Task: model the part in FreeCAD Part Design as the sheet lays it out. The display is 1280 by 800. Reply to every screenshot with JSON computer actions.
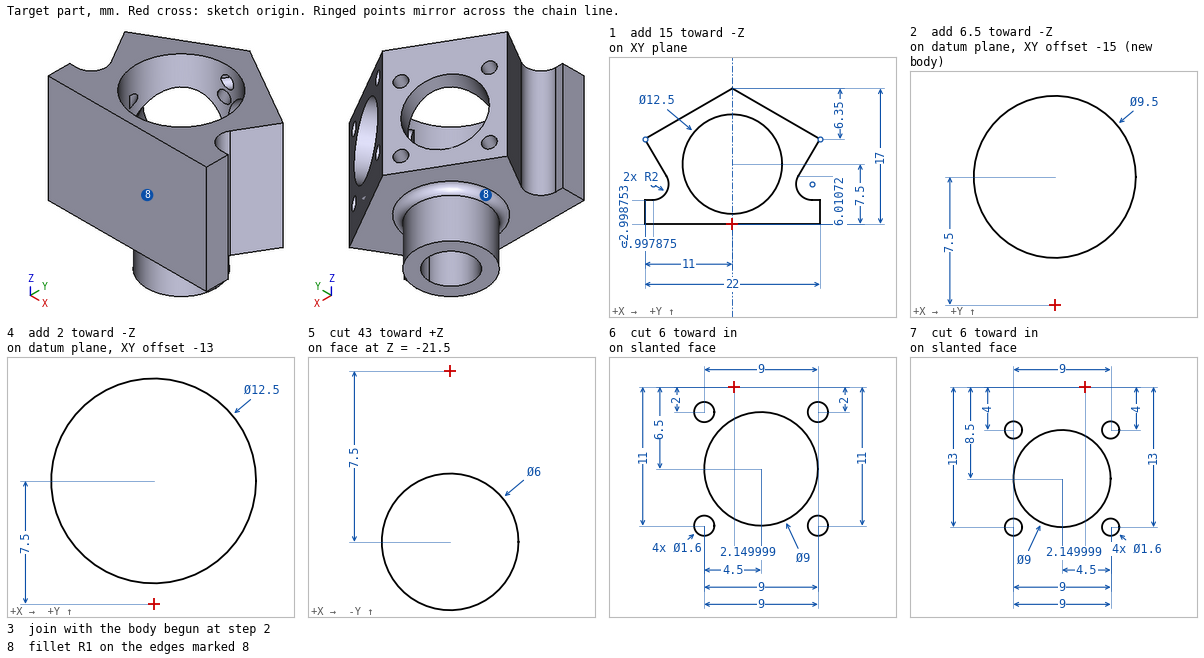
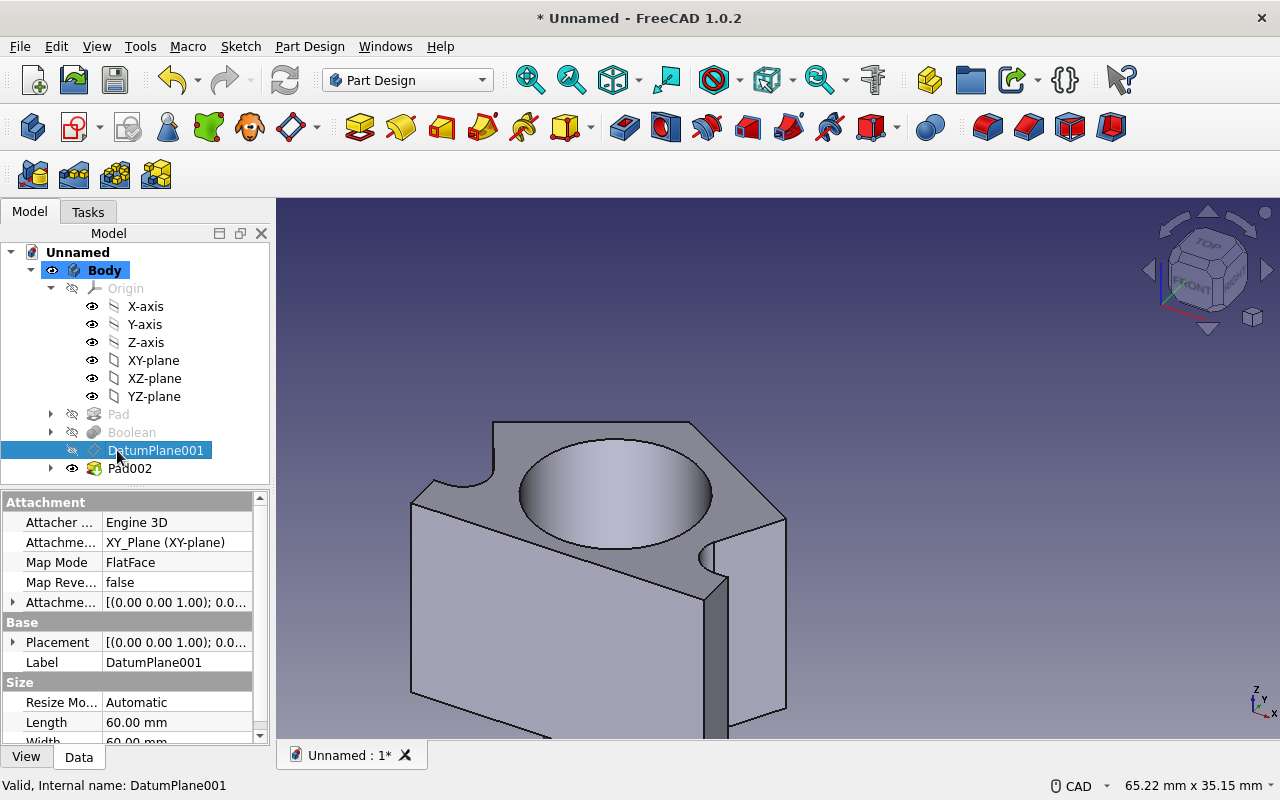
{"action": "left_click", "coordinate": [531, 80]}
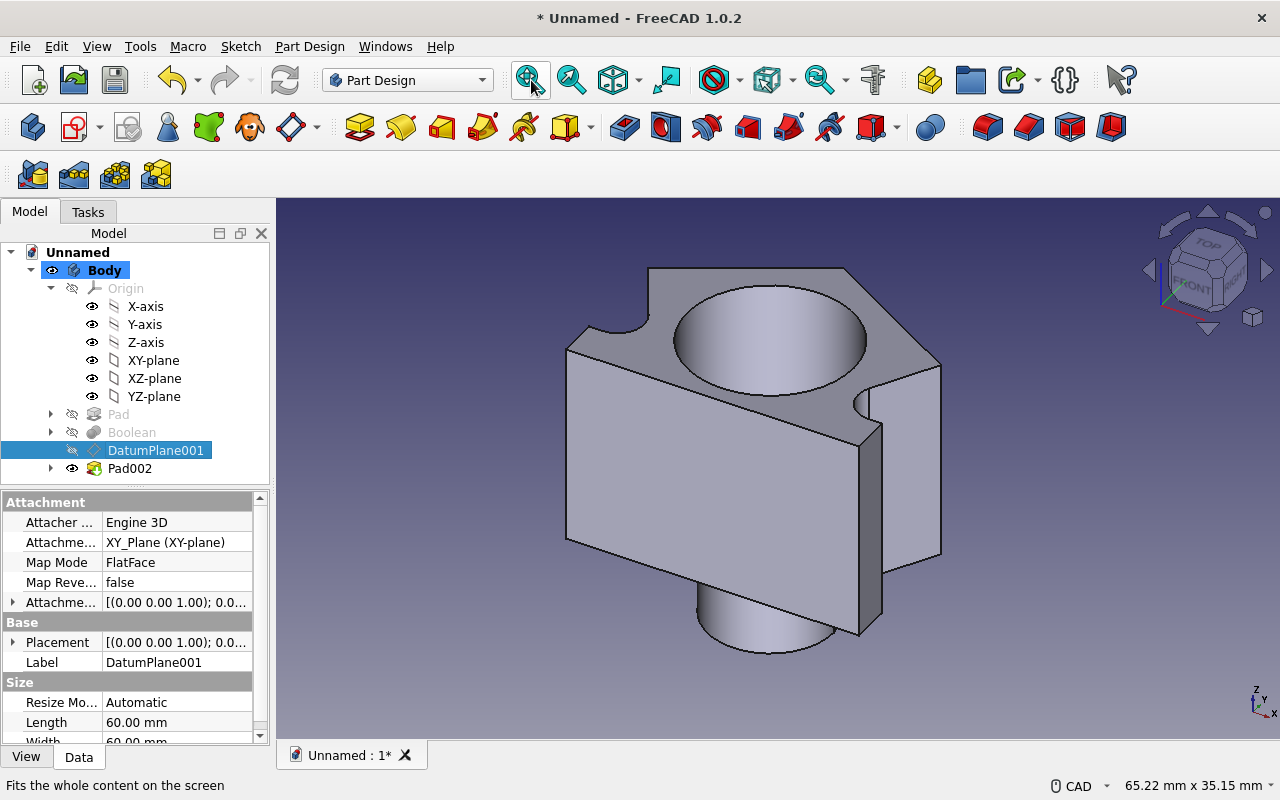
{"action": "key", "text": "5"}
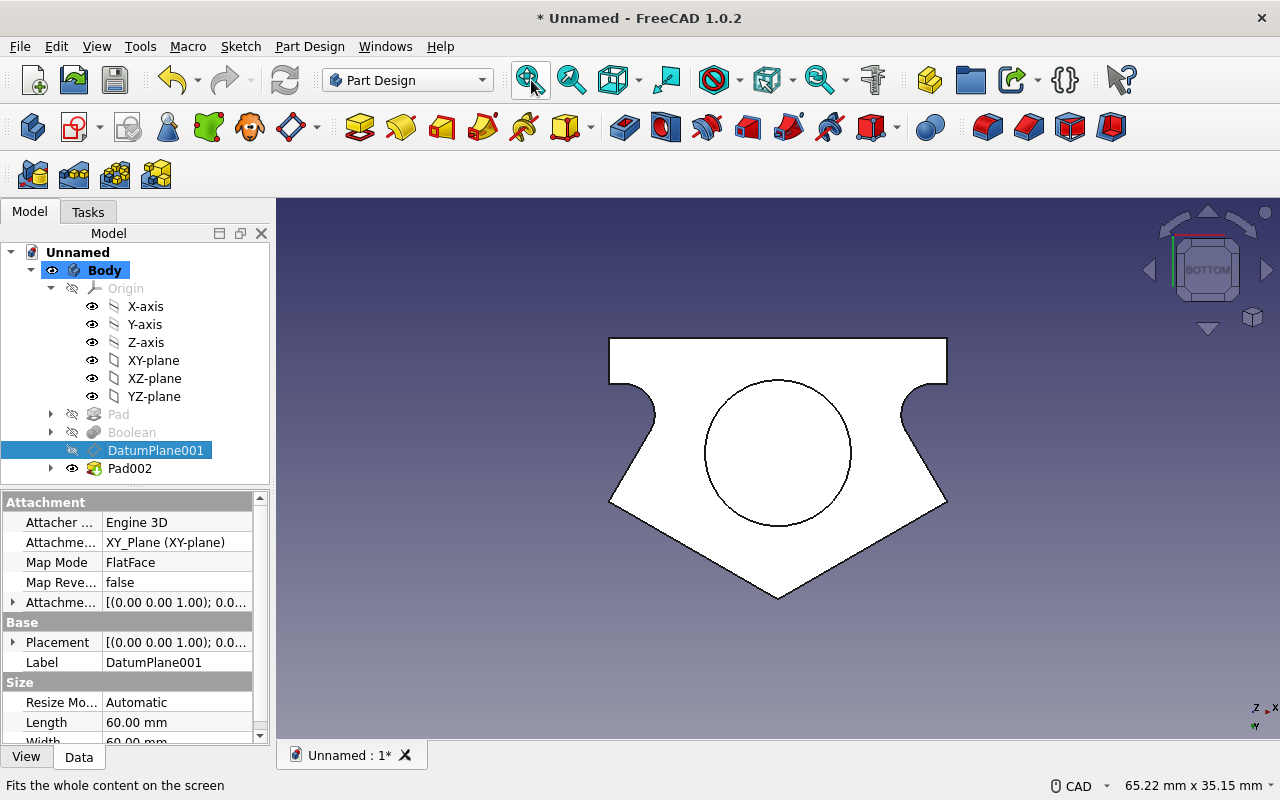
{"action": "left_click", "coordinate": [778, 452]}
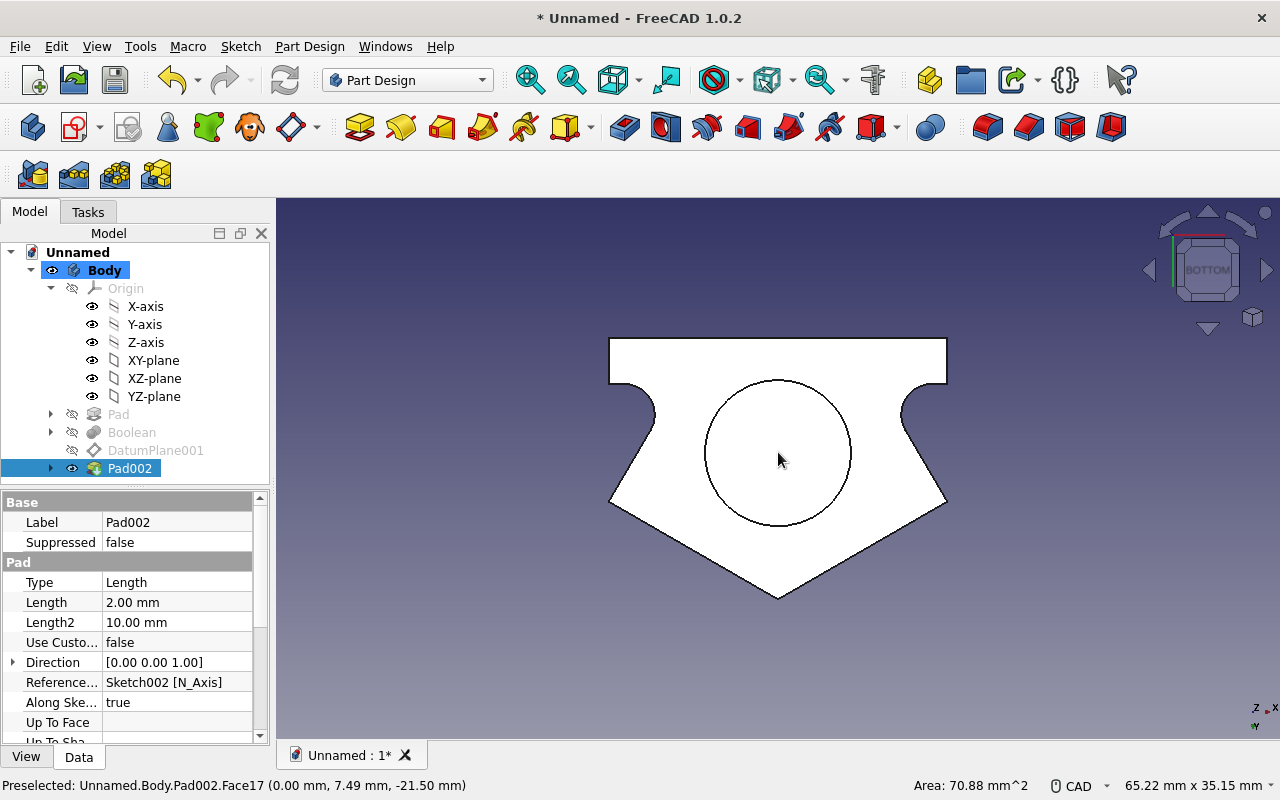
{"action": "left_click", "coordinate": [74, 128]}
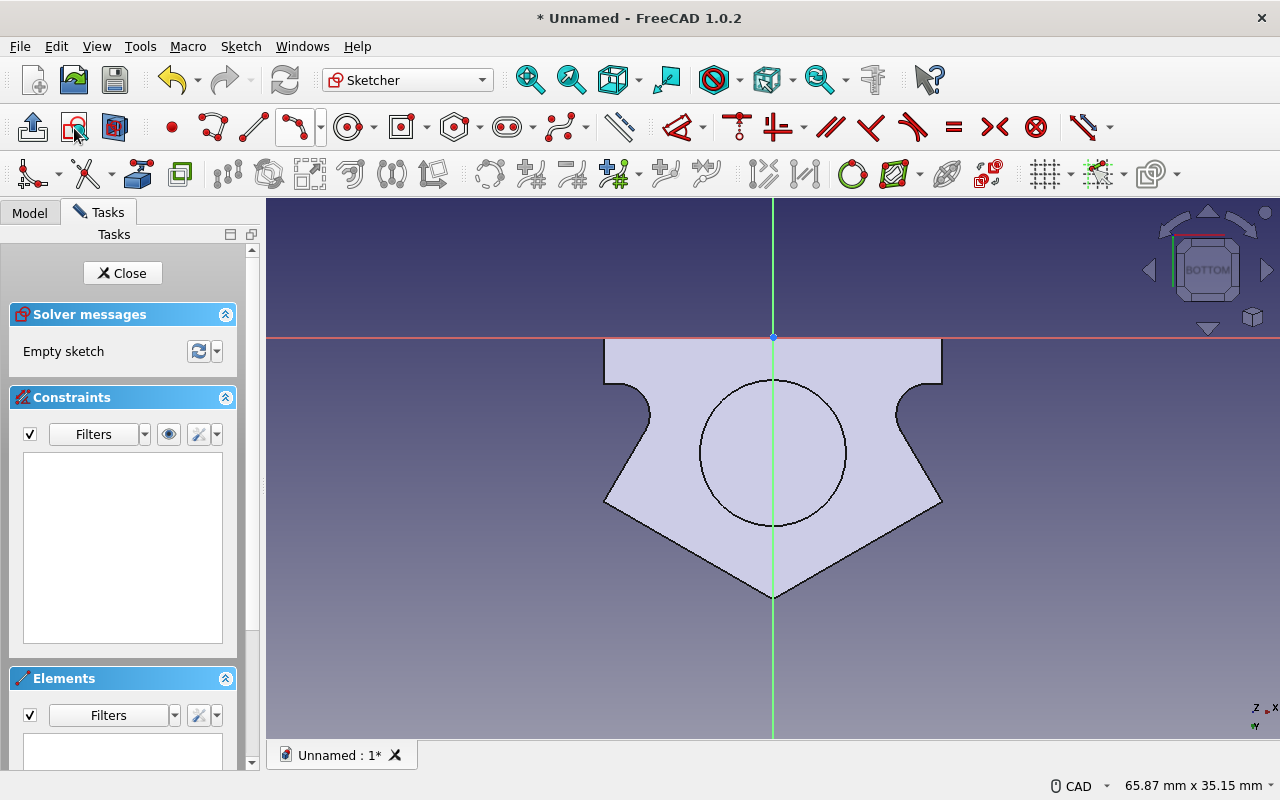
{"action": "scroll", "coordinate": [829, 378], "scroll_direction": "up", "scroll_amount": 4}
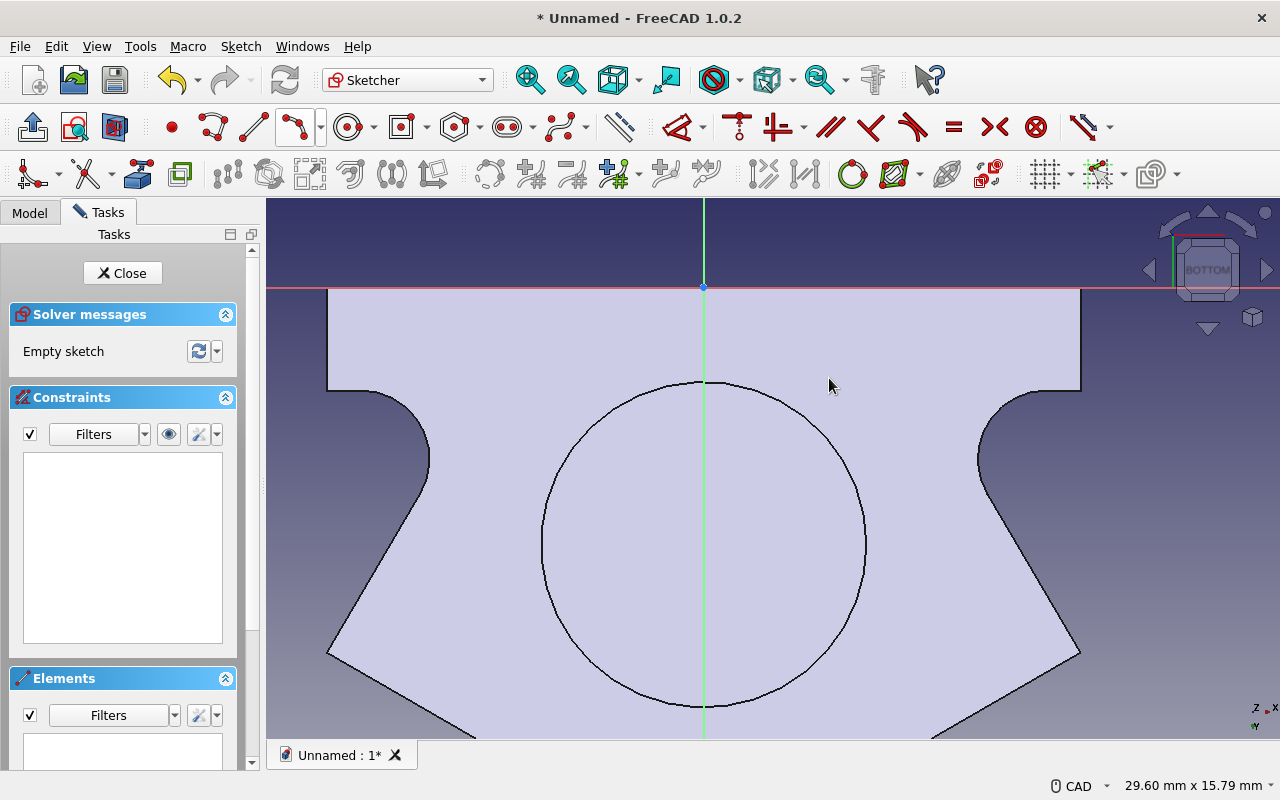
{"action": "left_click", "coordinate": [348, 128]}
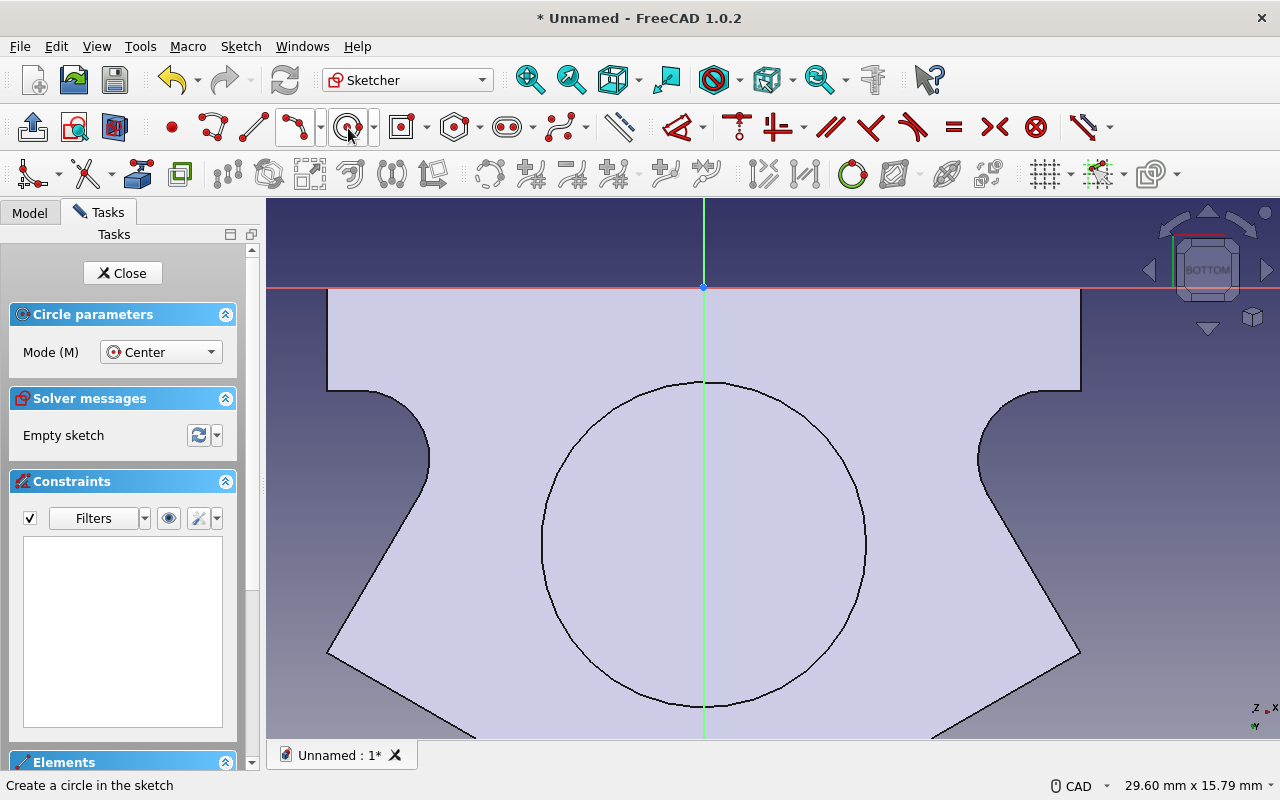
{"action": "left_click", "coordinate": [704, 545]}
{"action": "mouse_move", "coordinate": [776, 472]}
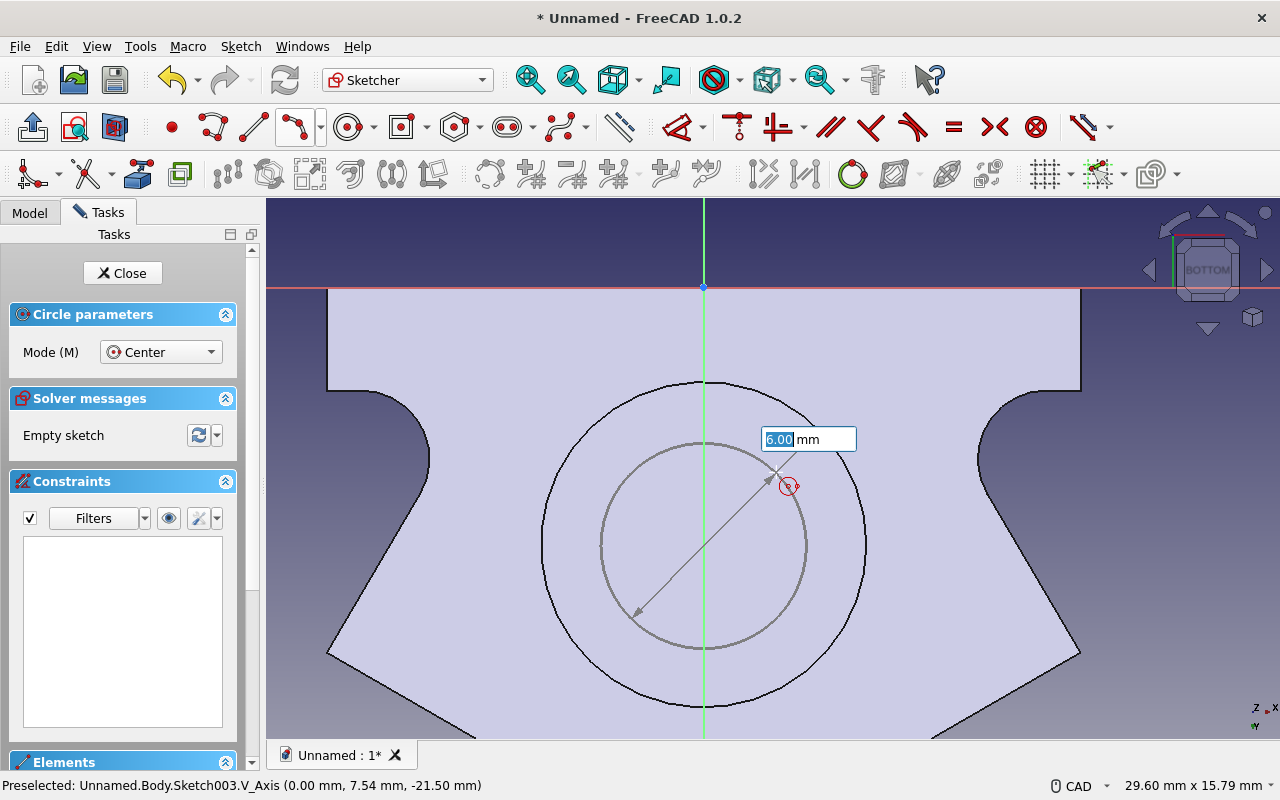
{"action": "type", "text": "6"}
{"action": "key", "text": "Return"}
{"action": "key", "text": "Escape"}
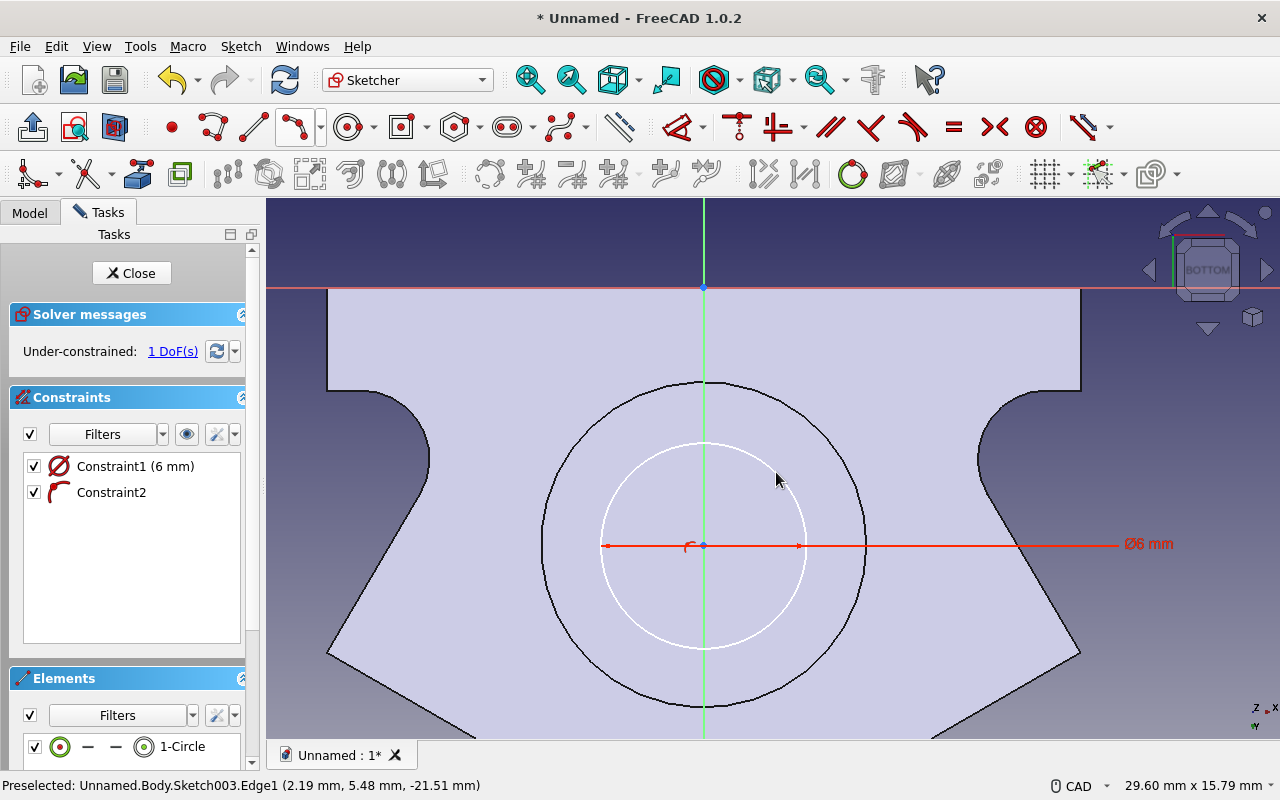
{"action": "left_click", "coordinate": [676, 128]}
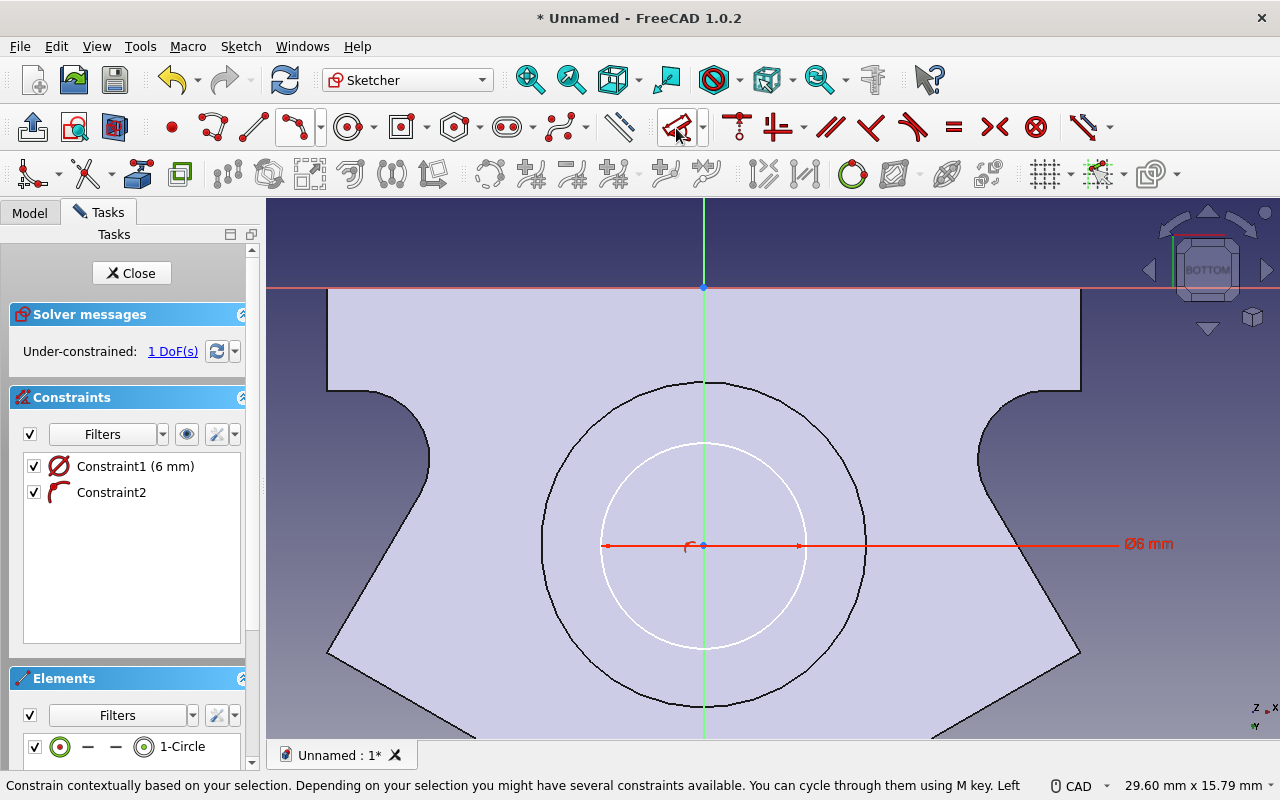
{"action": "left_click", "coordinate": [704, 546]}
{"action": "left_click", "coordinate": [738, 417]}